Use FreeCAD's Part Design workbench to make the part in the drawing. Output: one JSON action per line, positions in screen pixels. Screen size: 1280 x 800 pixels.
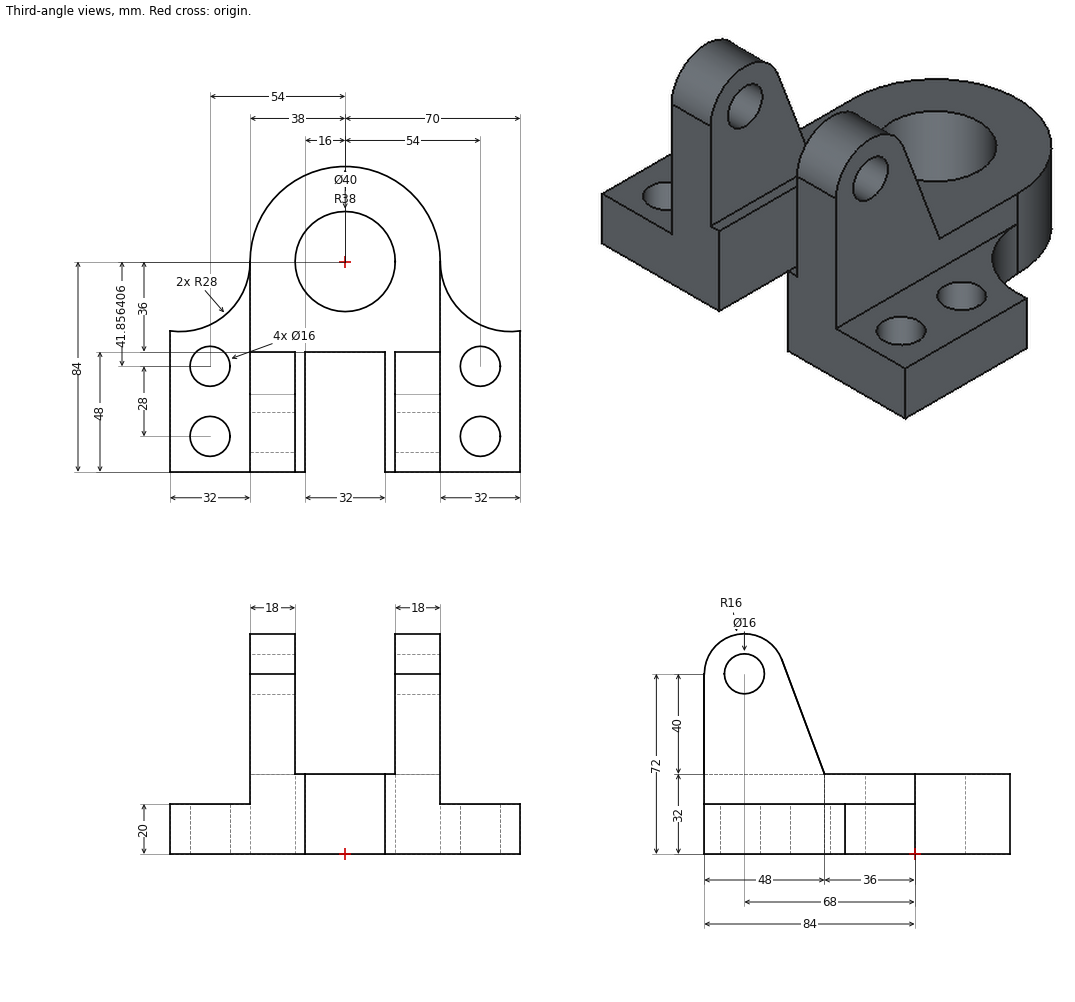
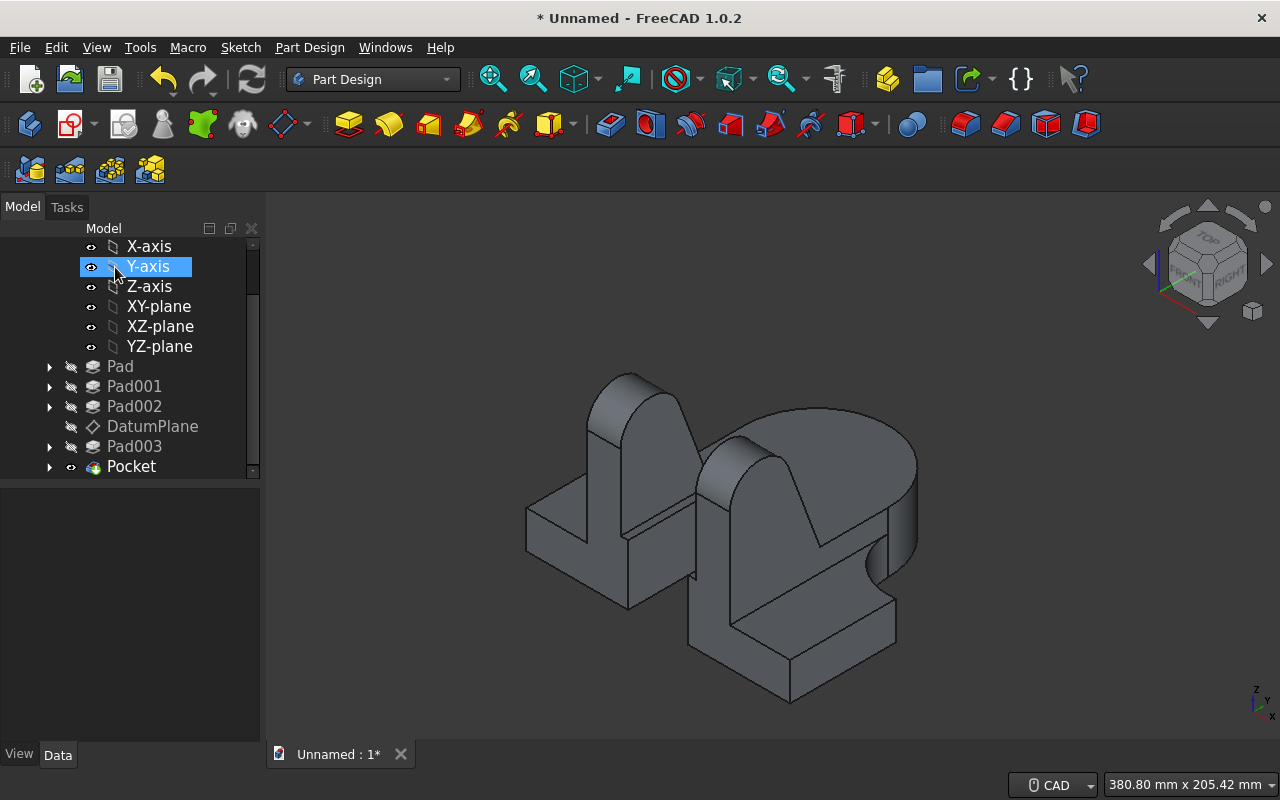
{"action": "left_click", "coordinate": [816, 609]}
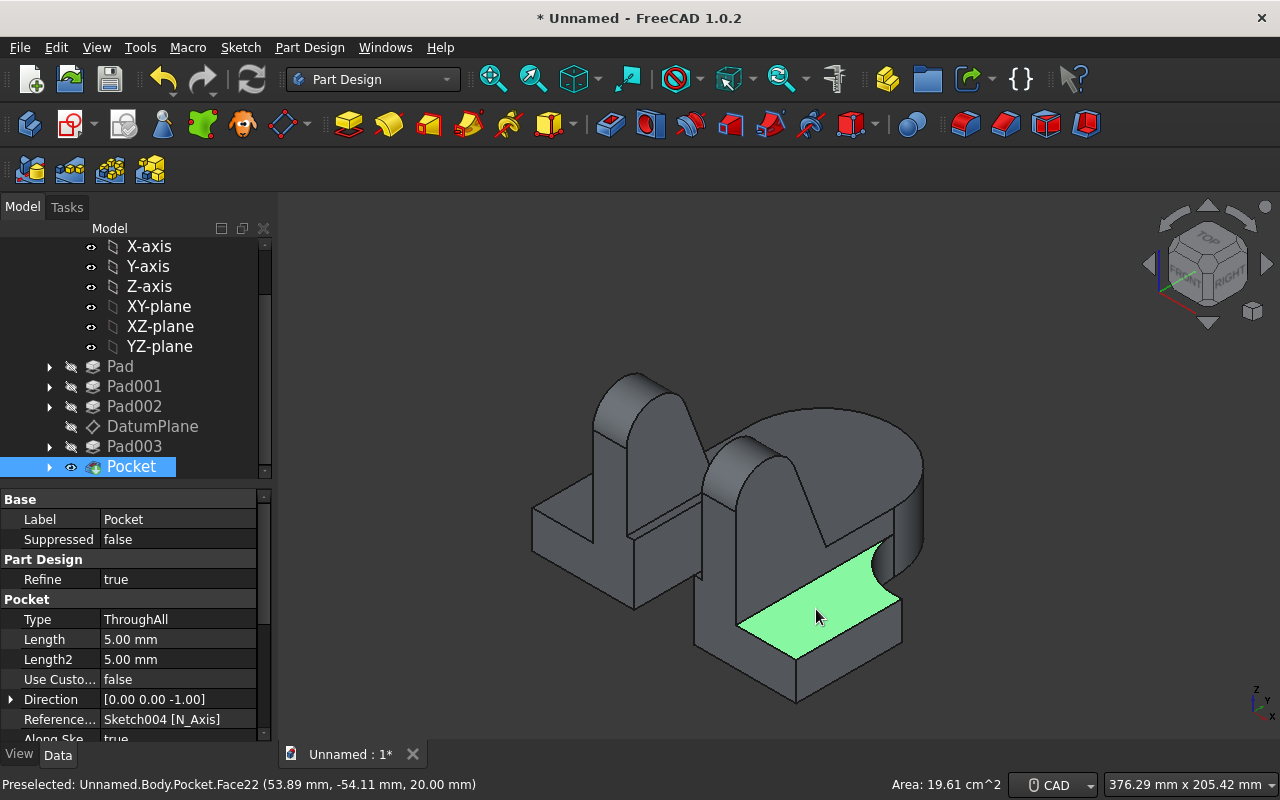
{"action": "left_click", "coordinate": [70, 124]}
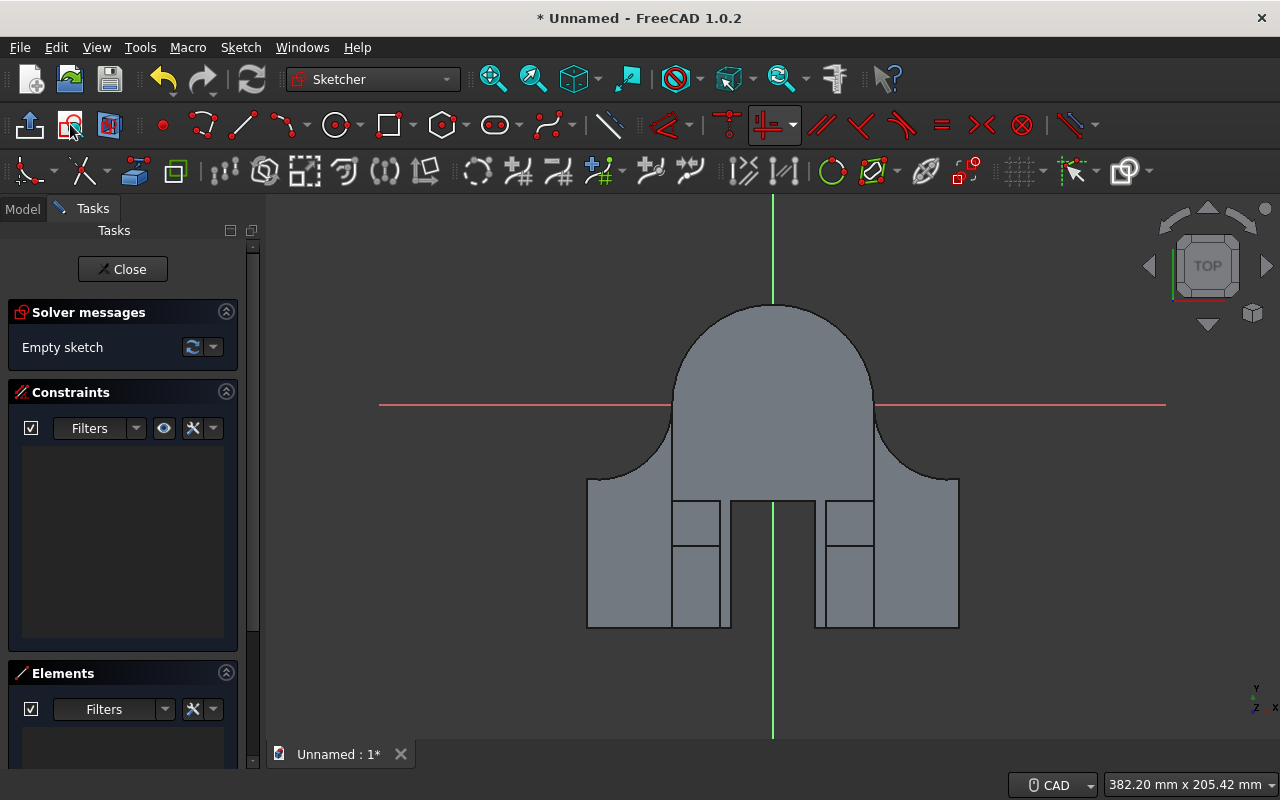
{"action": "left_click", "coordinate": [110, 126]}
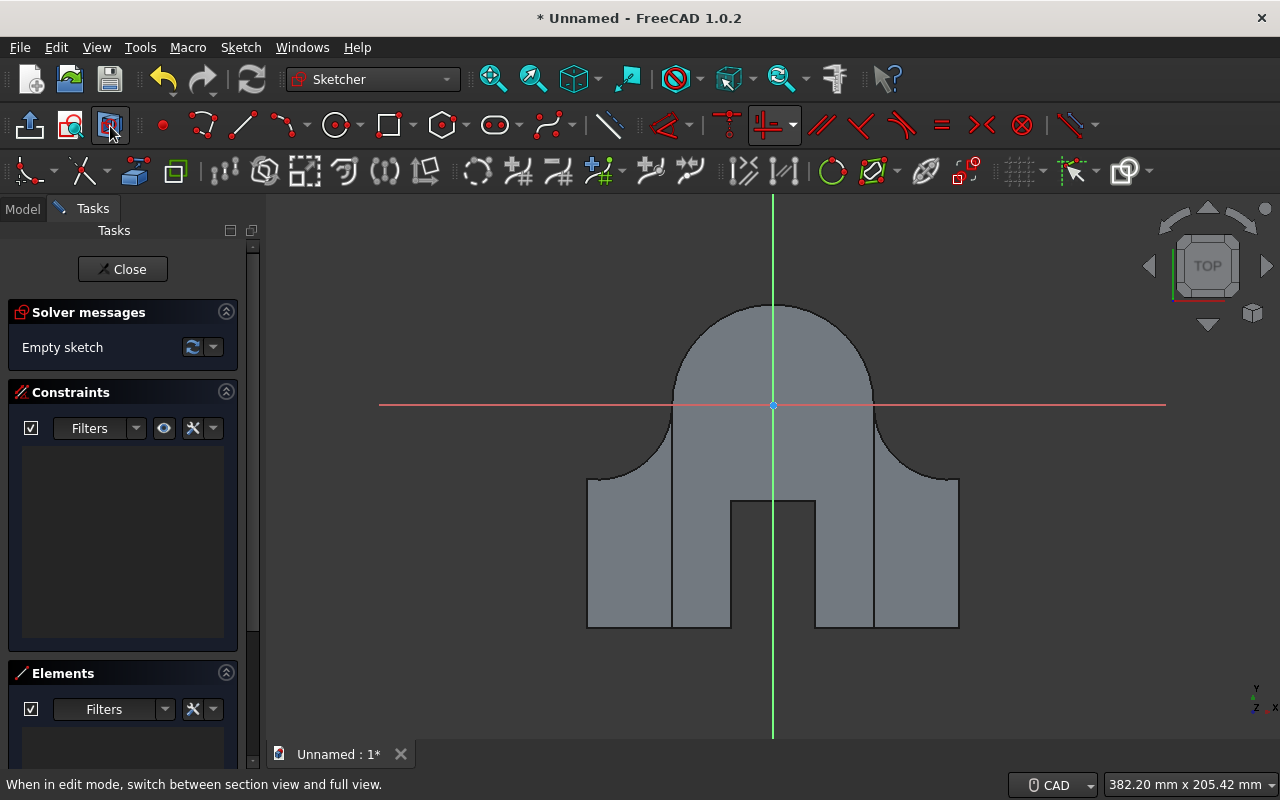
{"action": "scroll", "coordinate": [856, 560], "scroll_direction": "up", "scroll_amount": 3}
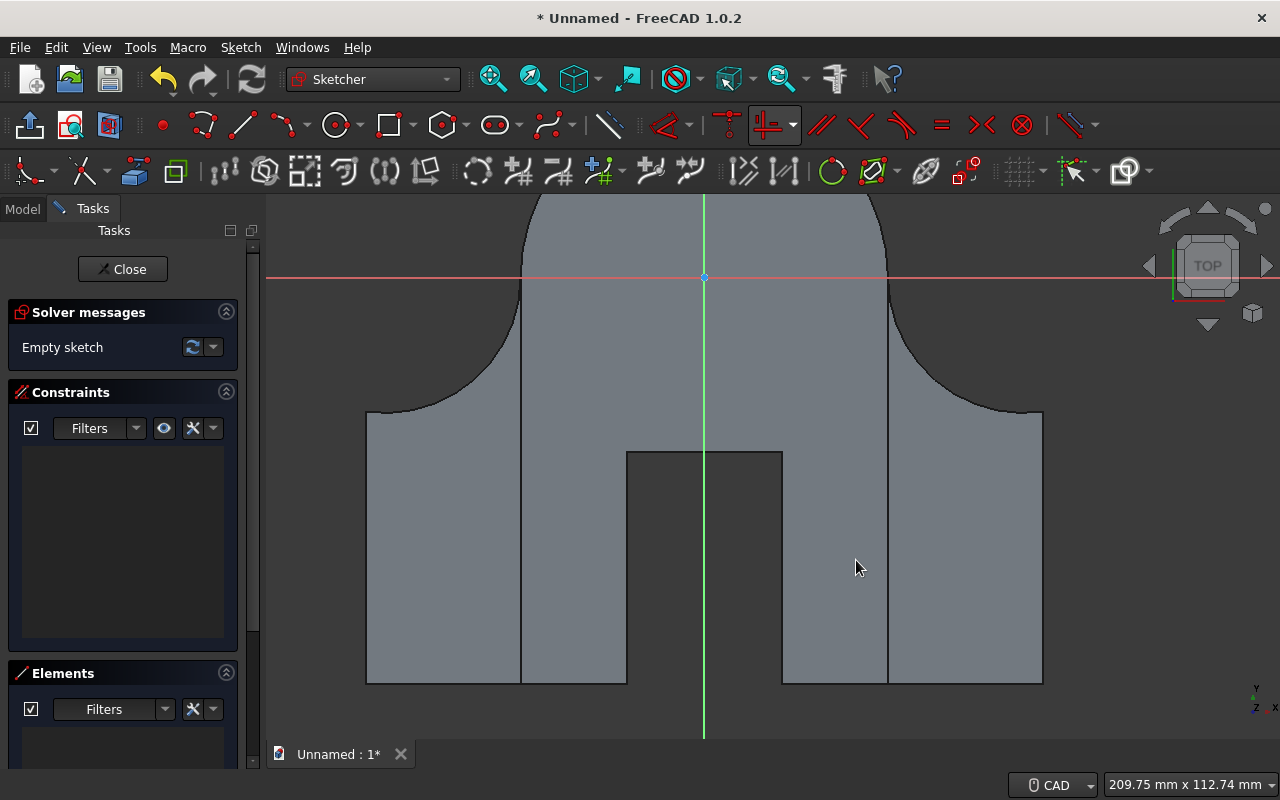
{"action": "left_click", "coordinate": [336, 126]}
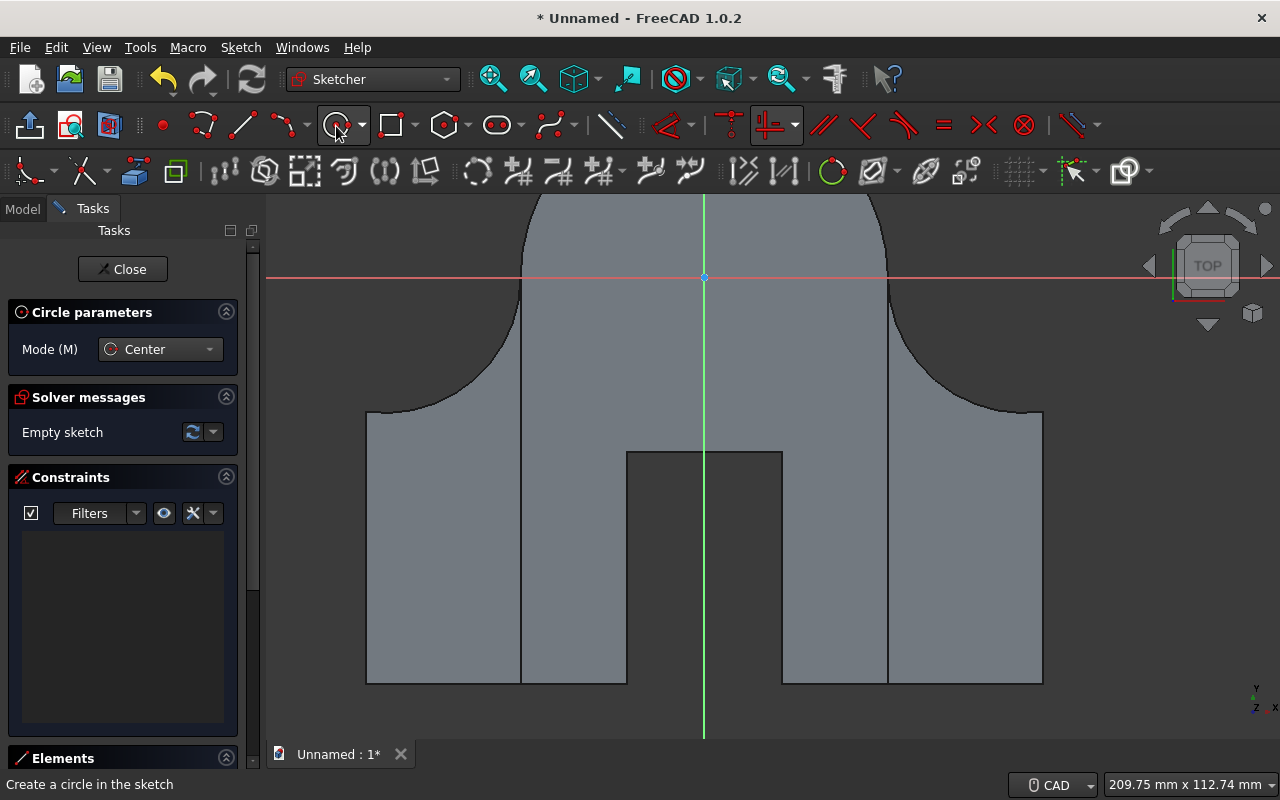
{"action": "left_click", "coordinate": [443, 480]}
{"action": "left_click", "coordinate": [471, 453]}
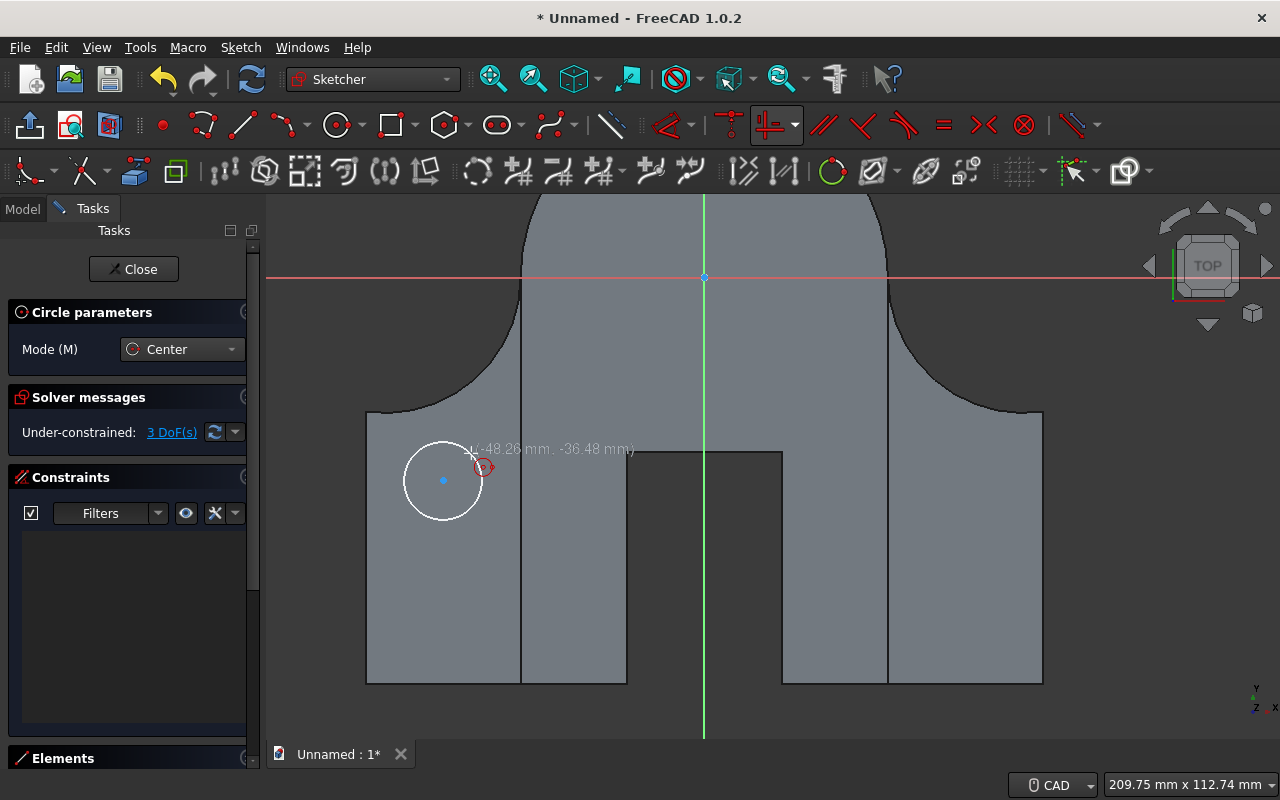
{"action": "left_click", "coordinate": [443, 615]}
{"action": "left_click", "coordinate": [471, 588]}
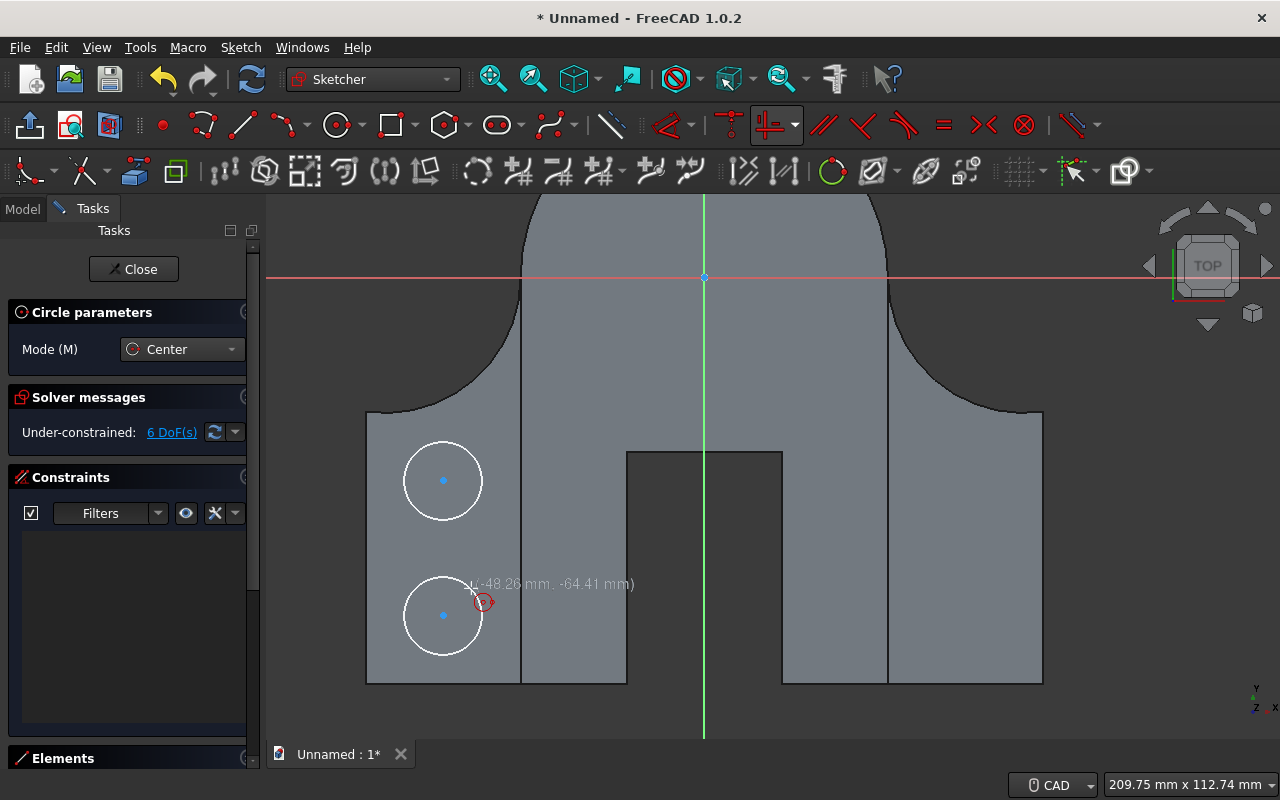
{"action": "left_click", "coordinate": [965, 480]}
{"action": "left_click", "coordinate": [993, 453]}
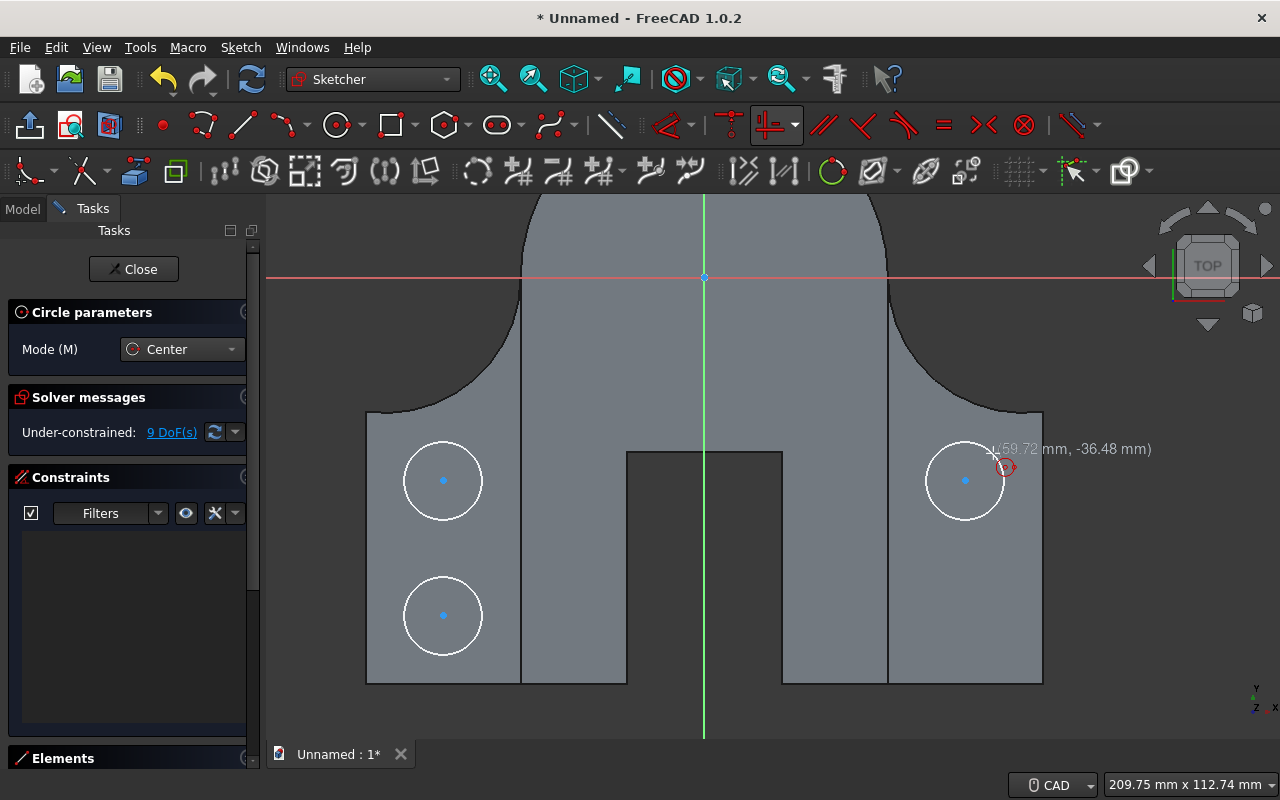
{"action": "left_click", "coordinate": [965, 615]}
{"action": "left_click", "coordinate": [993, 588]}
{"action": "key", "text": "Escape"}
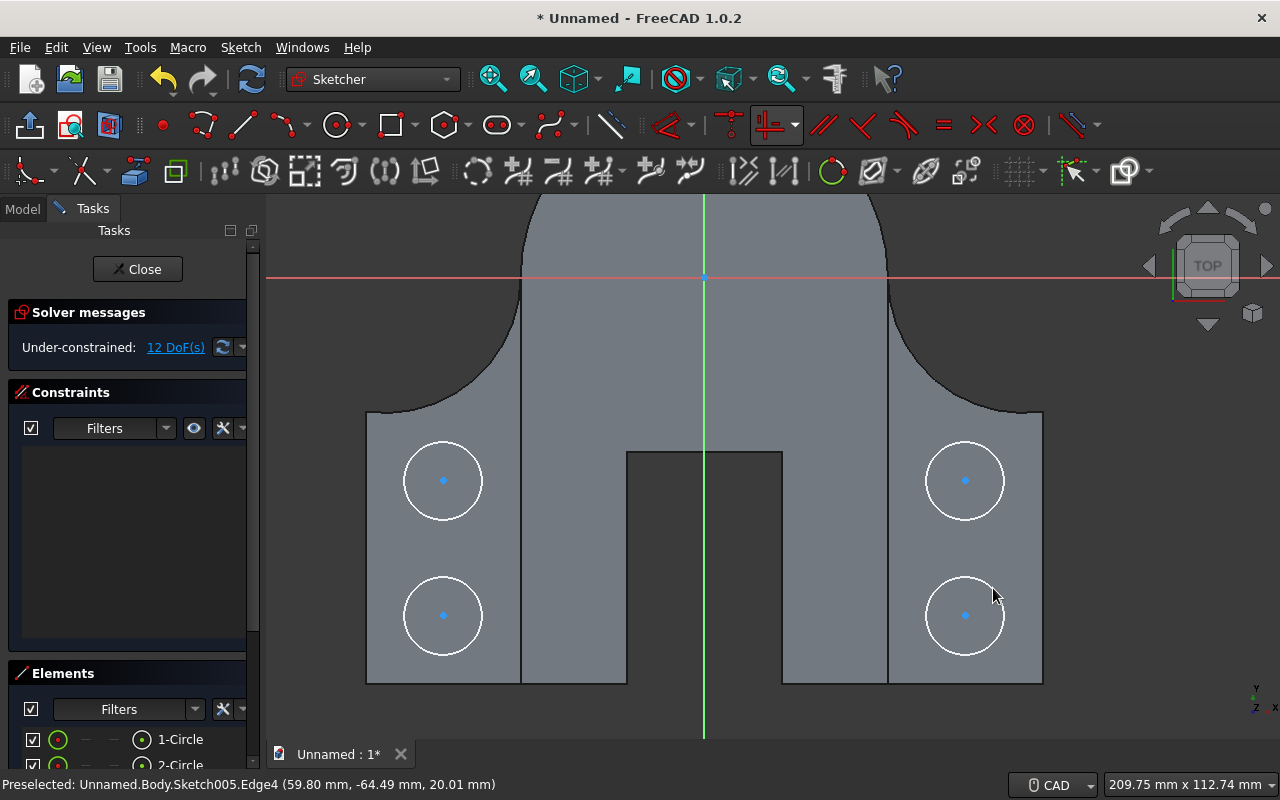
{"action": "left_click", "coordinate": [470, 453]}